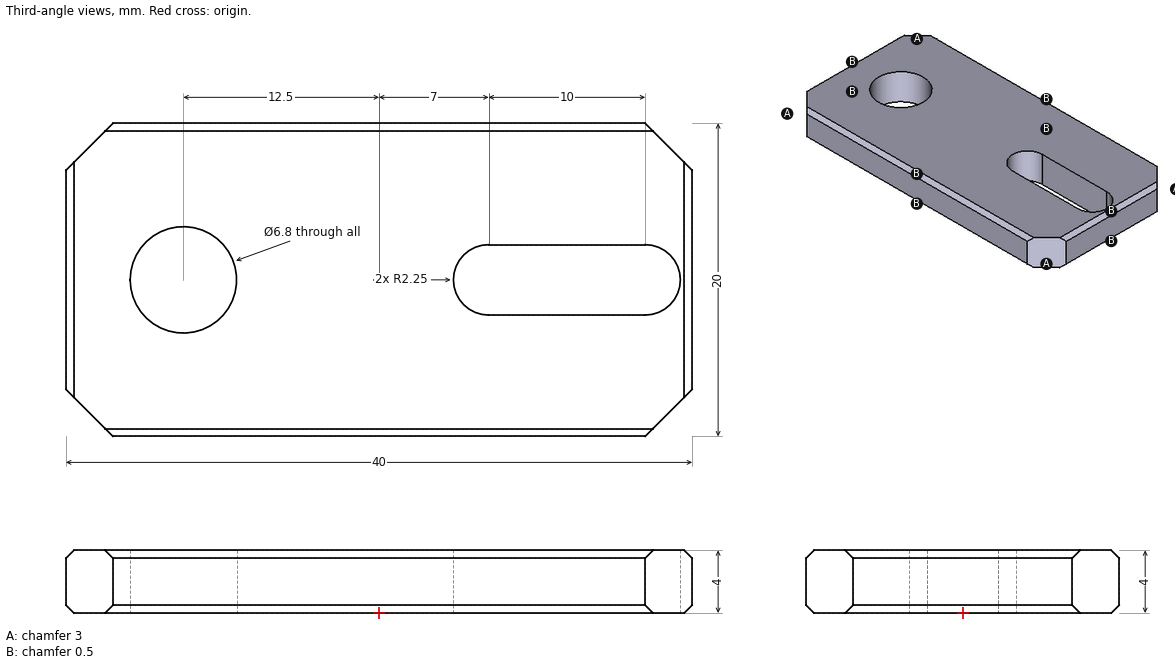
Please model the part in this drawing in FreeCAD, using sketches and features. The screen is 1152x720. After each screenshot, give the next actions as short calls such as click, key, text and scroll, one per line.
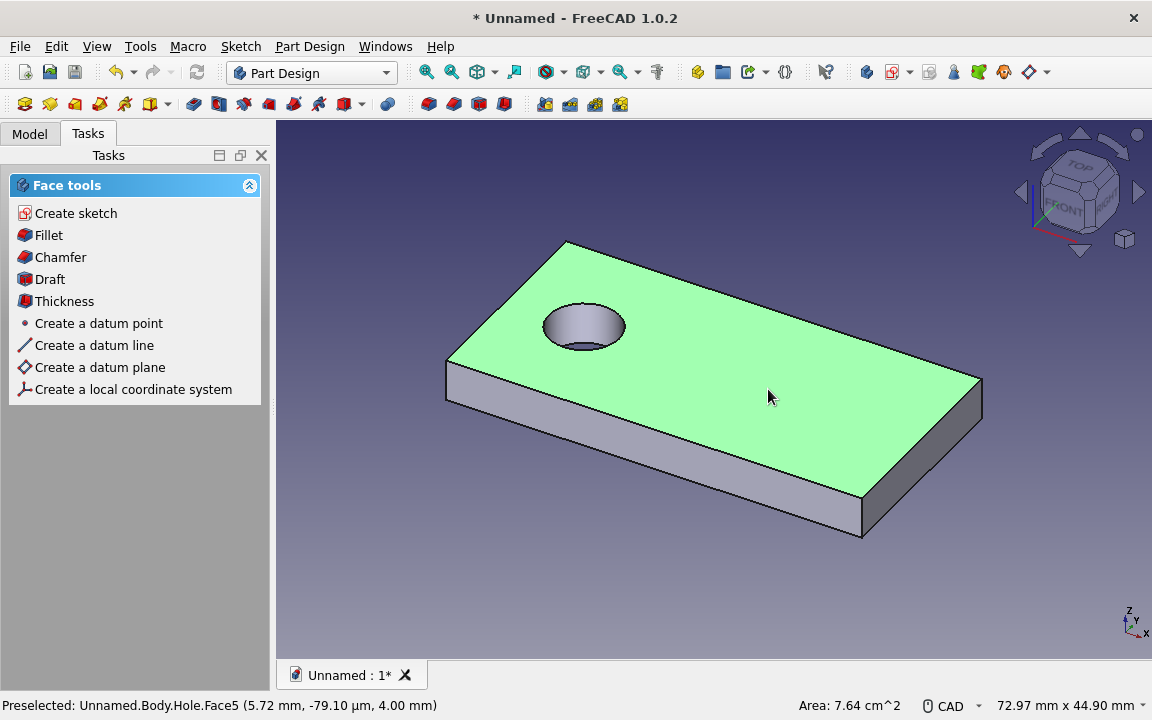
click(892, 72)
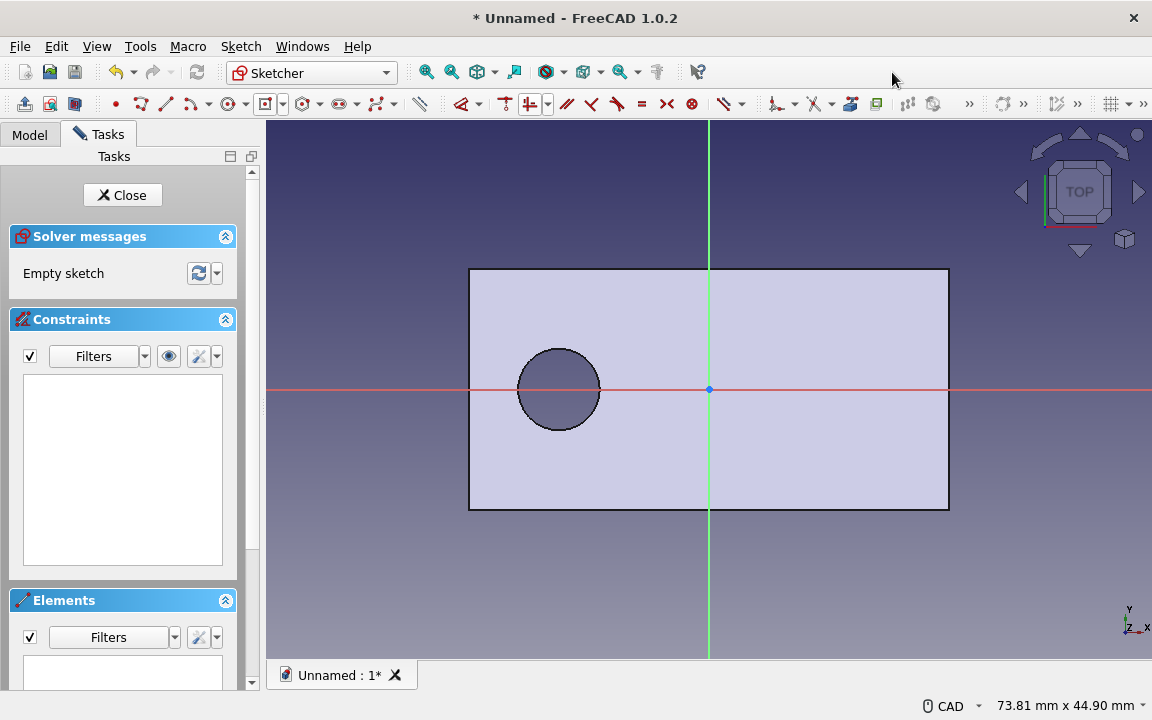
scroll(975, 390, up, 4)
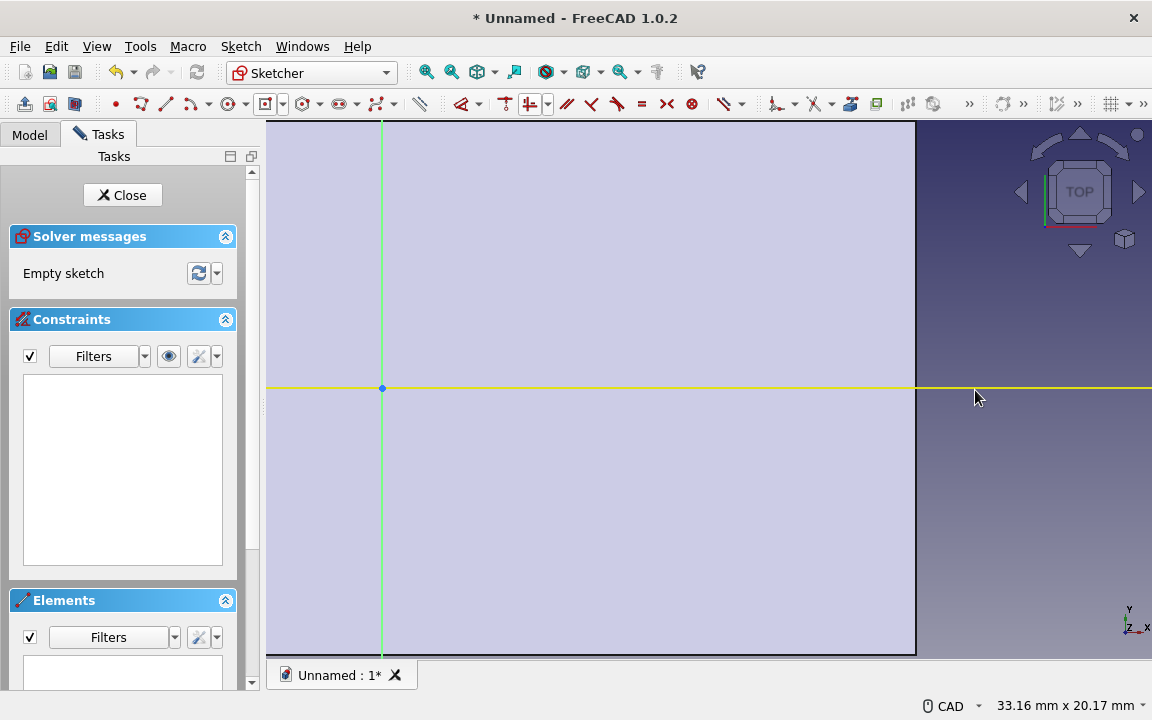
click(338, 104)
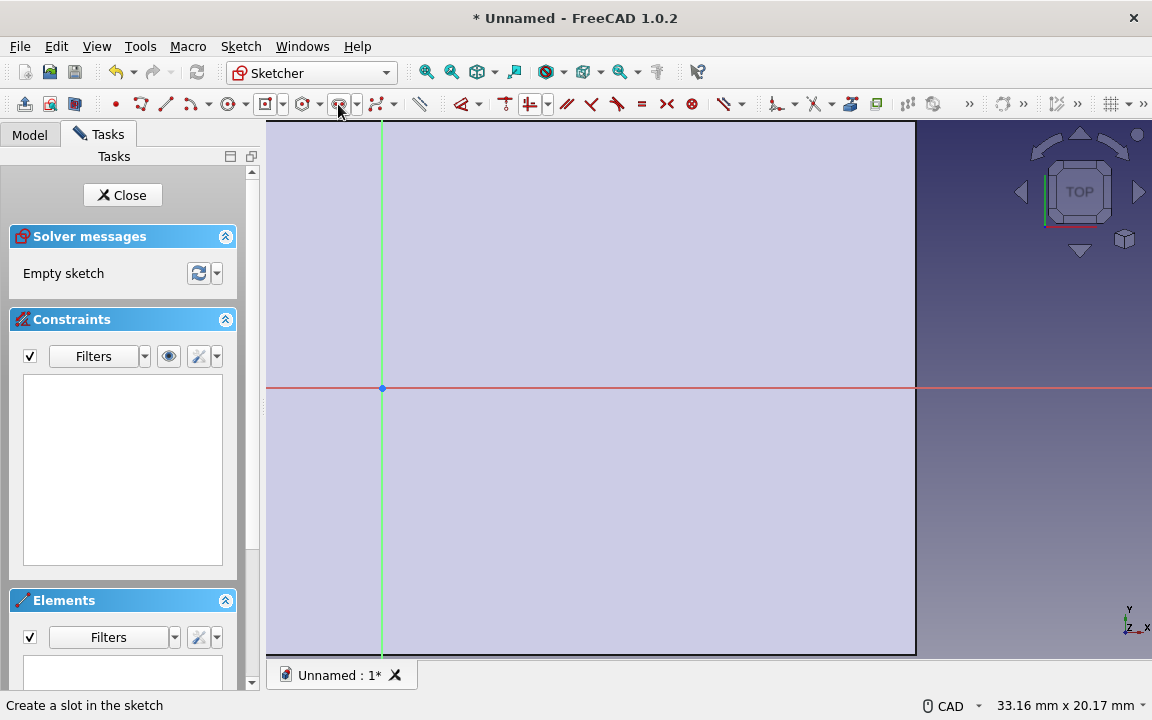
click(569, 388)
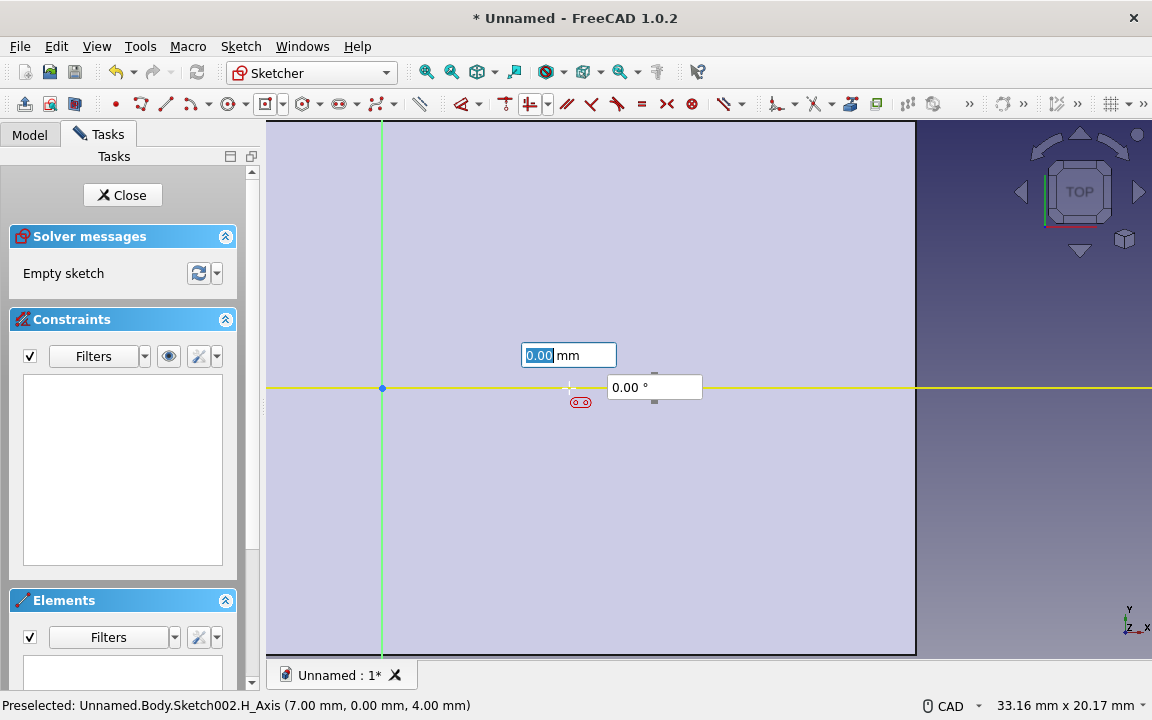
click(836, 379)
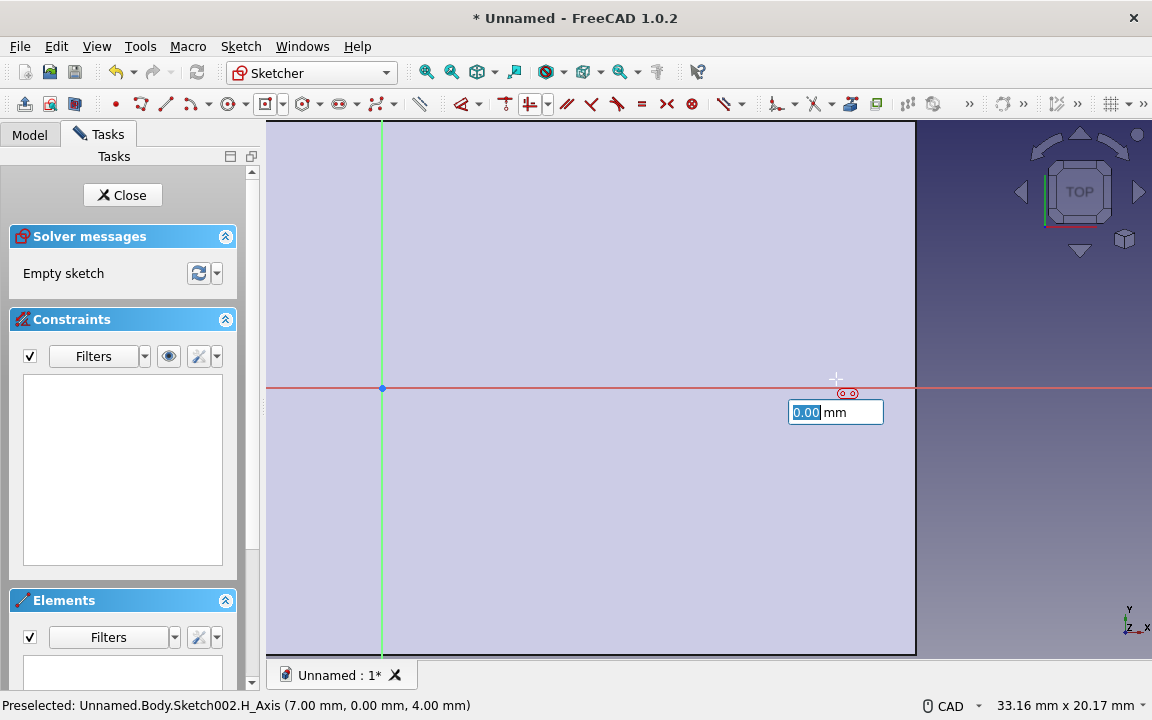
click(703, 328)
key(Escape)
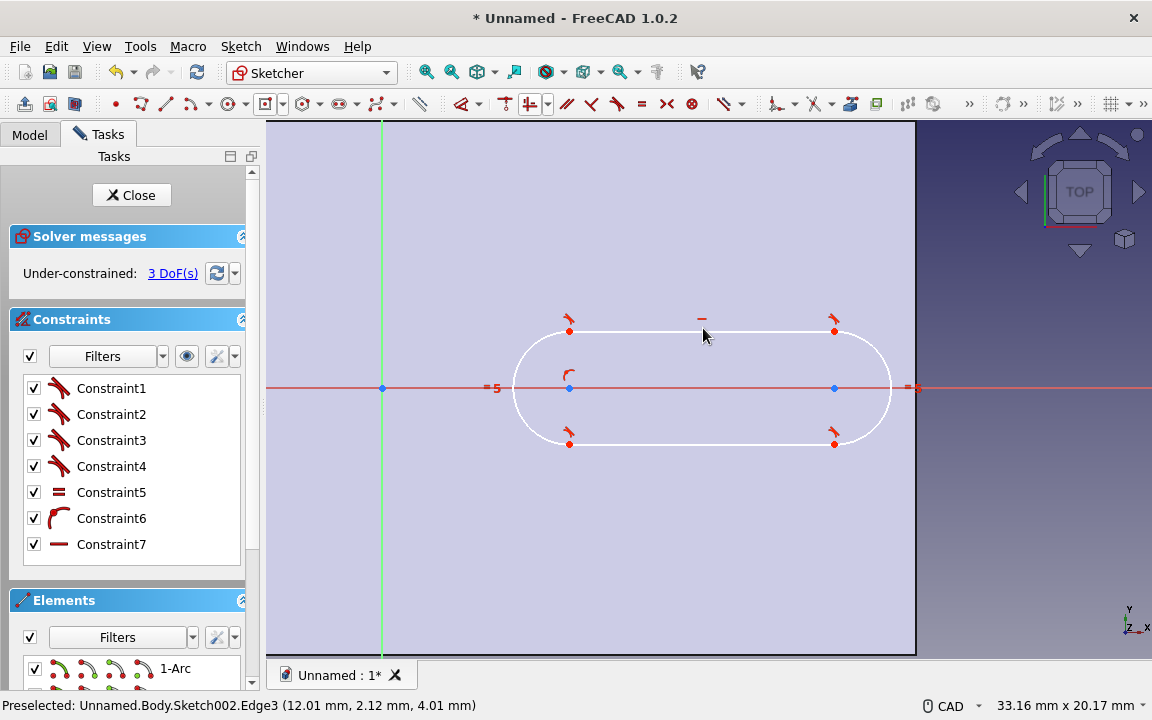
click(460, 104)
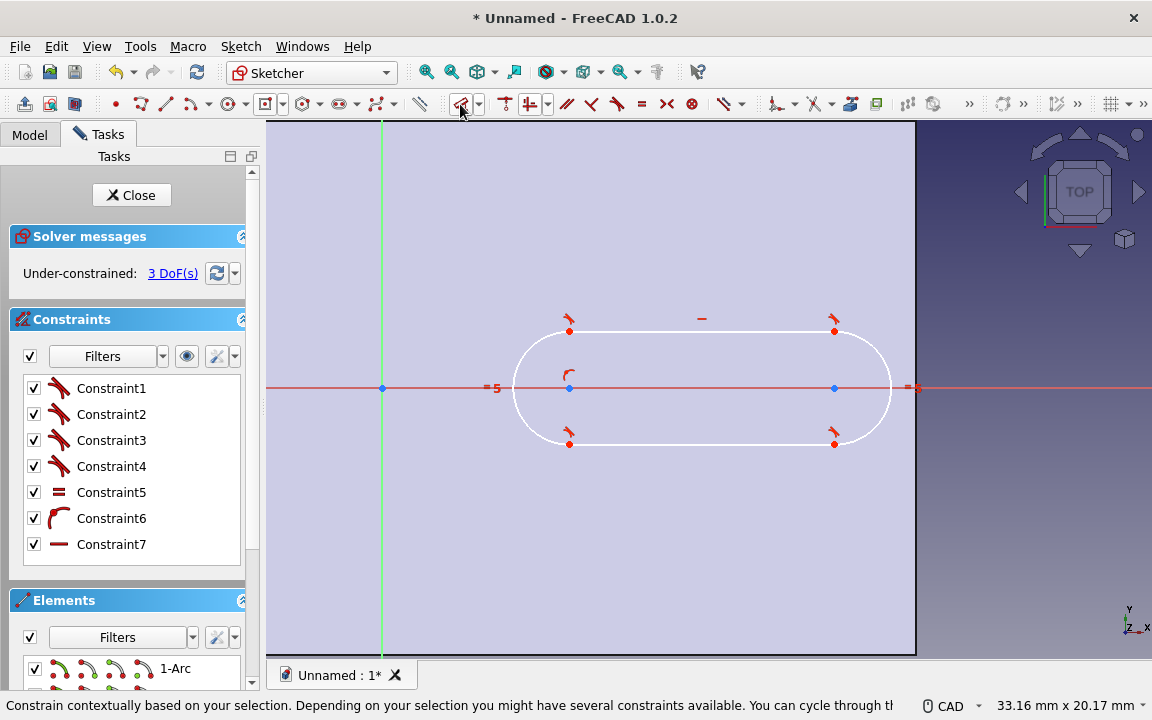
click(524, 355)
click(498, 336)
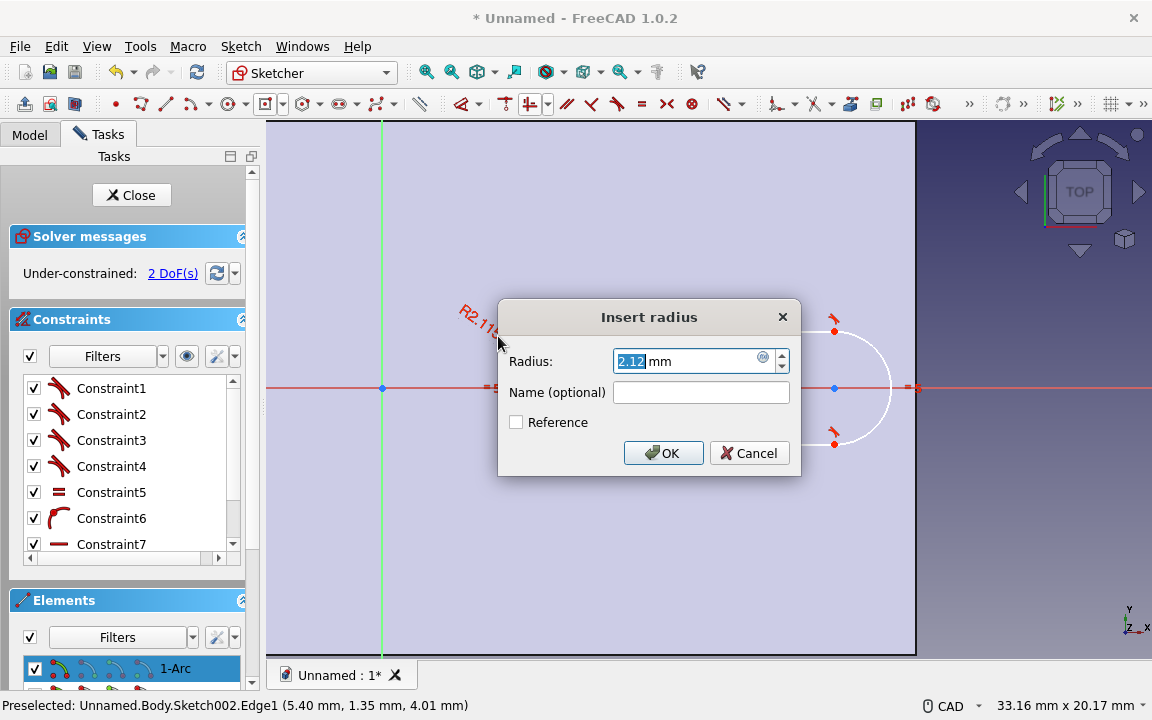
text(2.25)
key(Return)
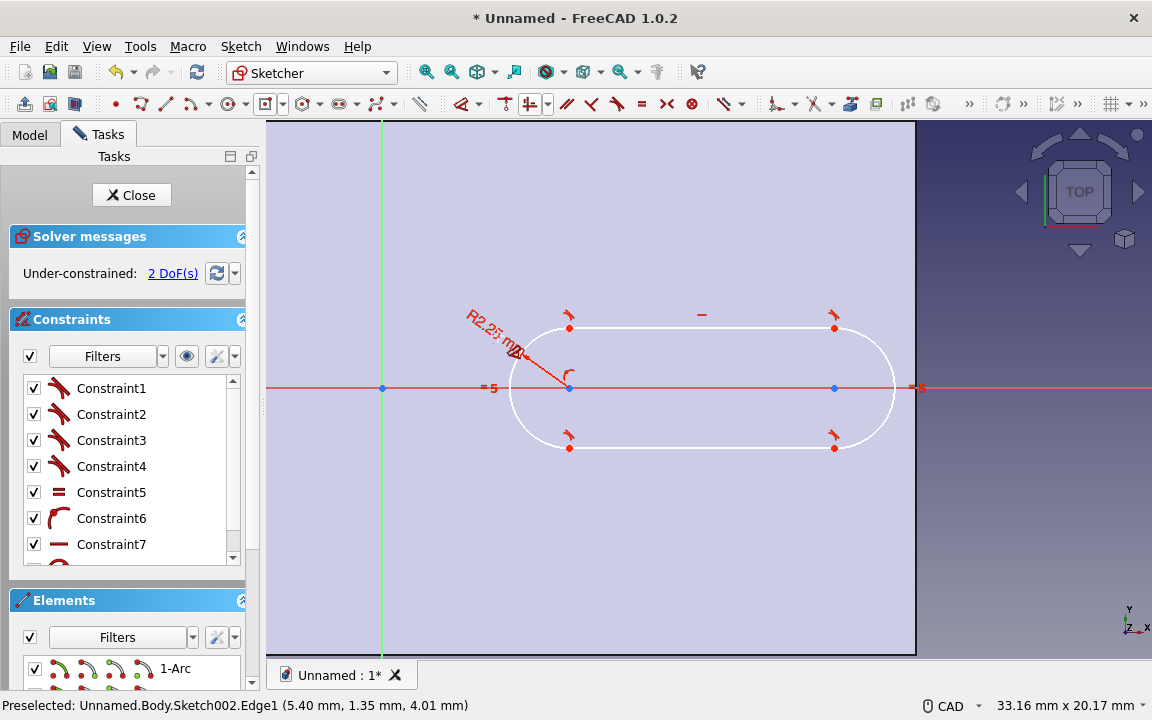
click(649, 328)
click(702, 294)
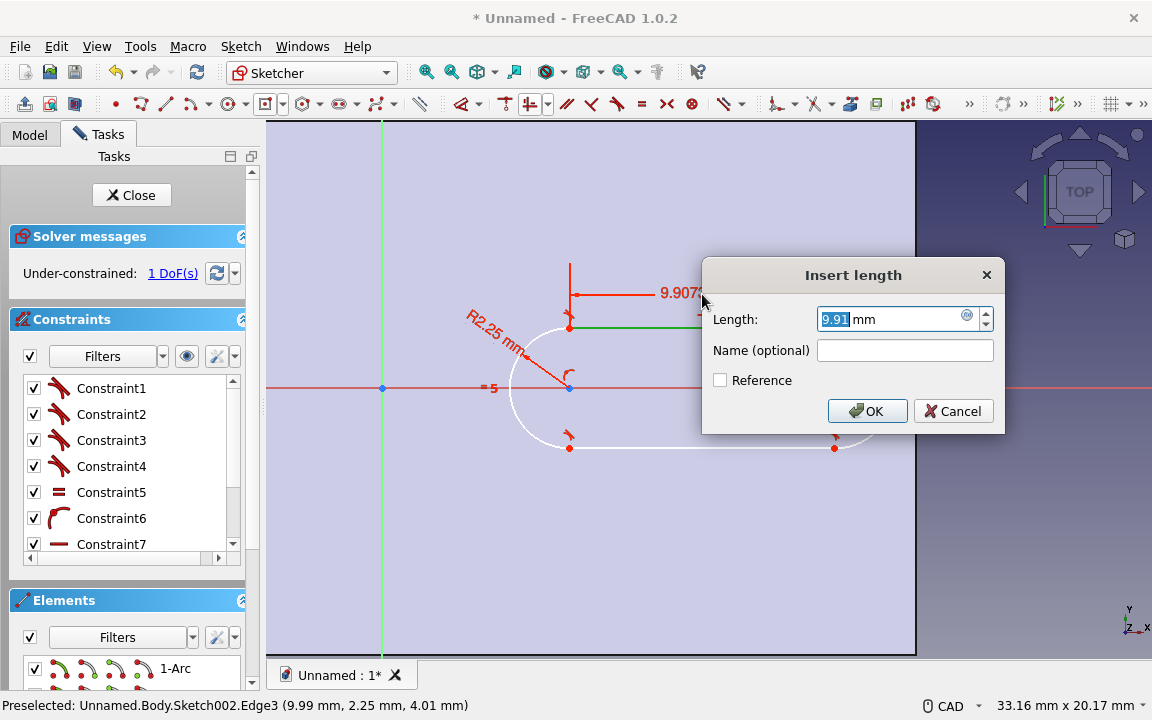
text(10)
key(Return)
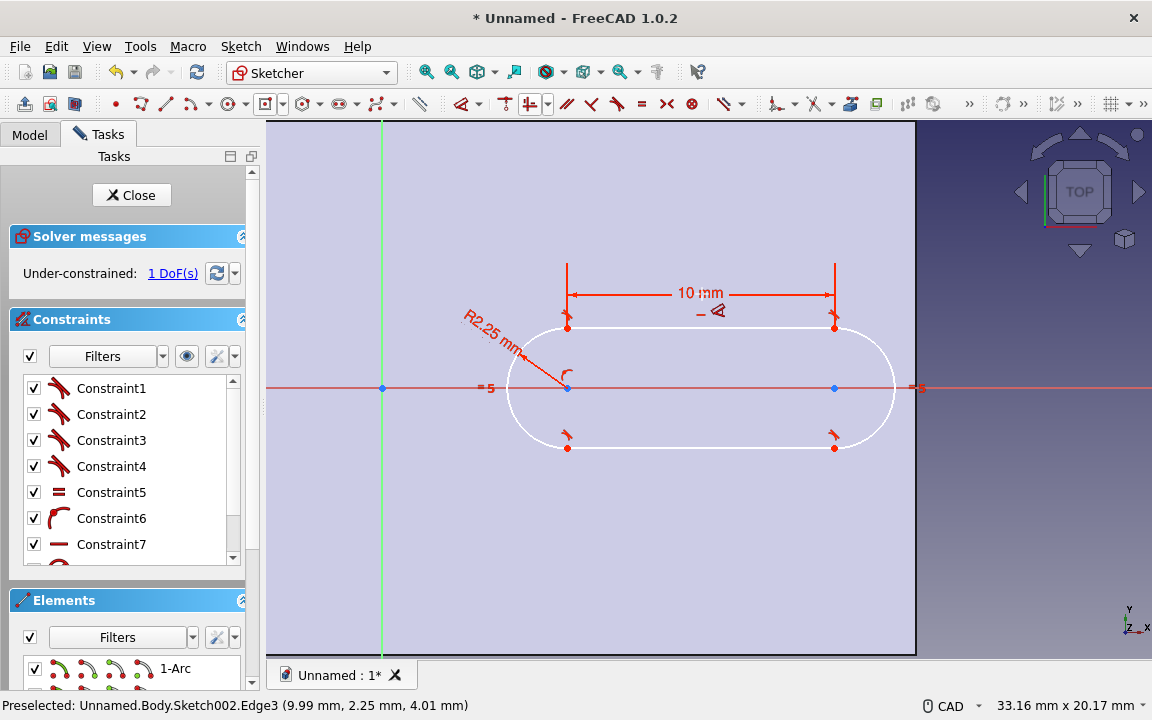
click(567, 328)
click(475, 294)